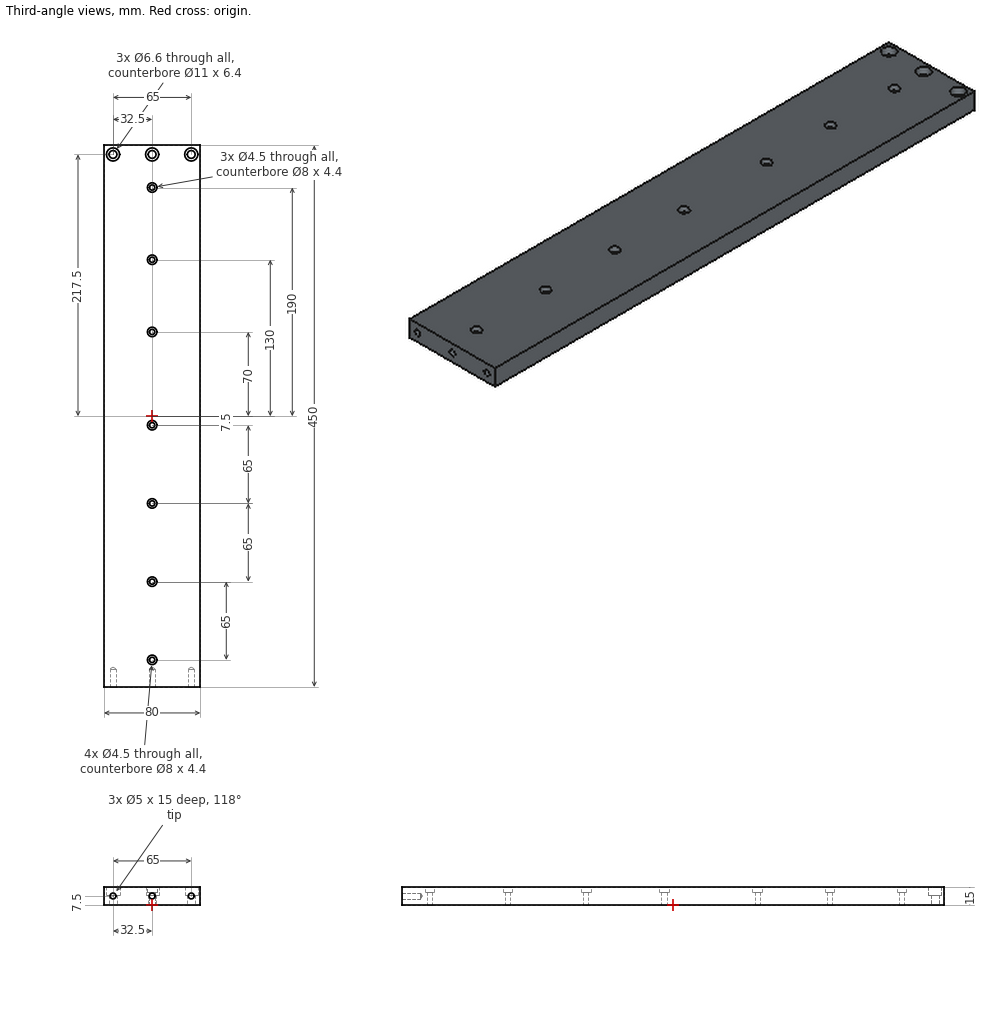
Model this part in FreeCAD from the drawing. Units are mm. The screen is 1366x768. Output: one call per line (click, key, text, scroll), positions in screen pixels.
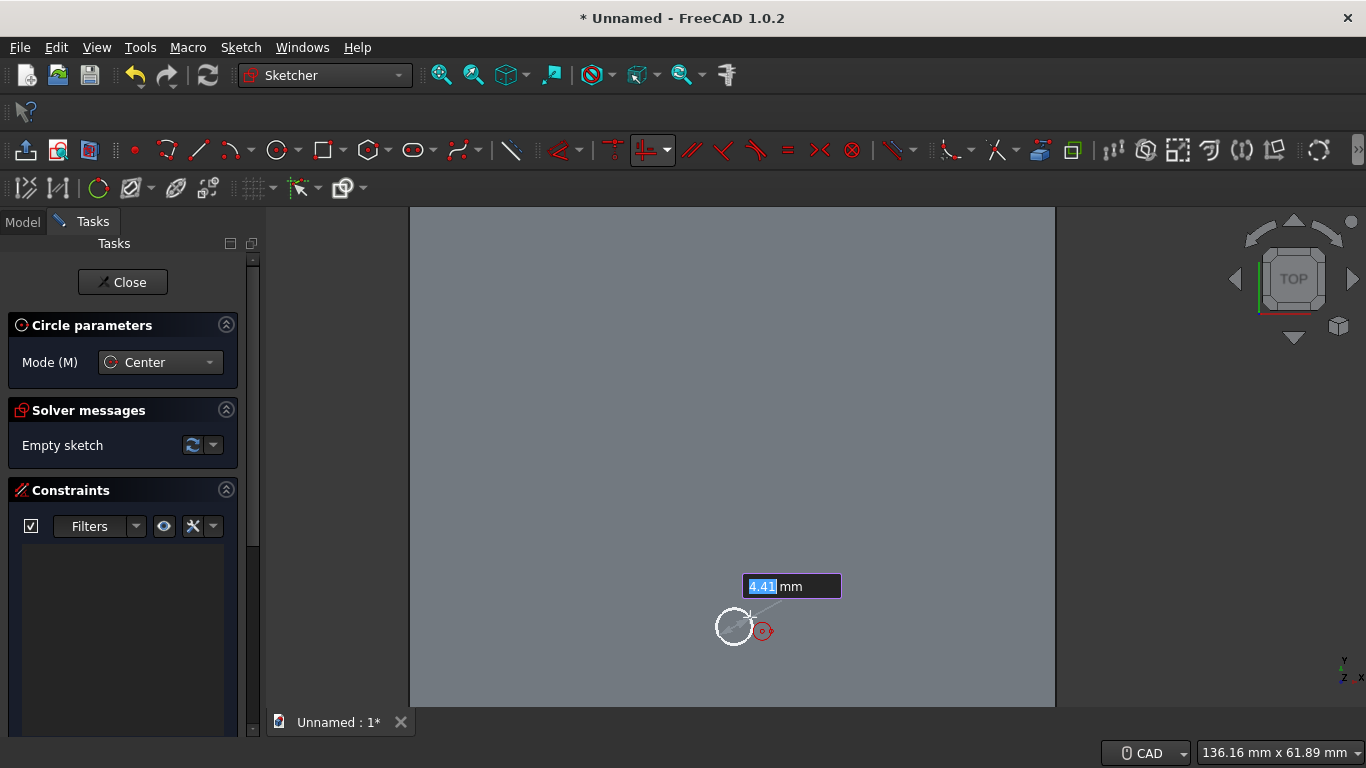
text(4.5)
key(Return)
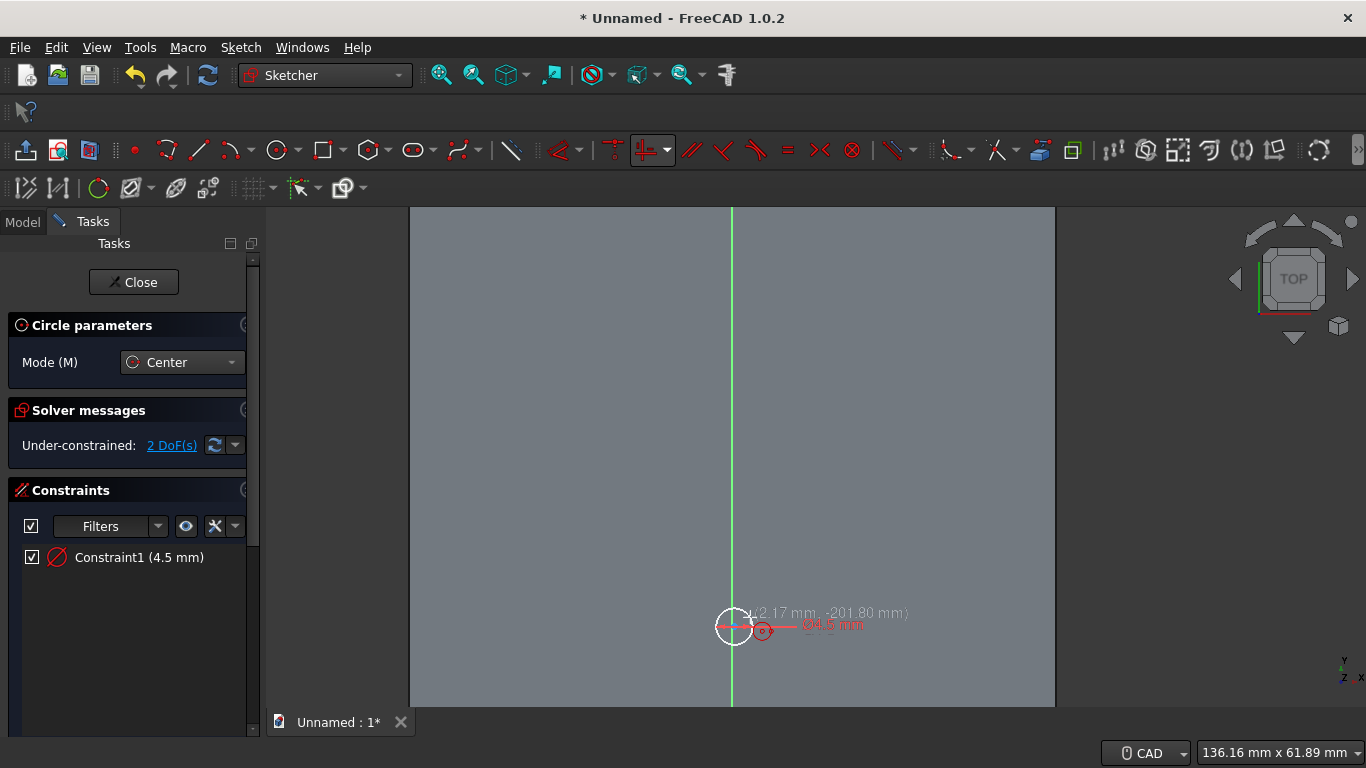
scroll(751, 619, down, 8)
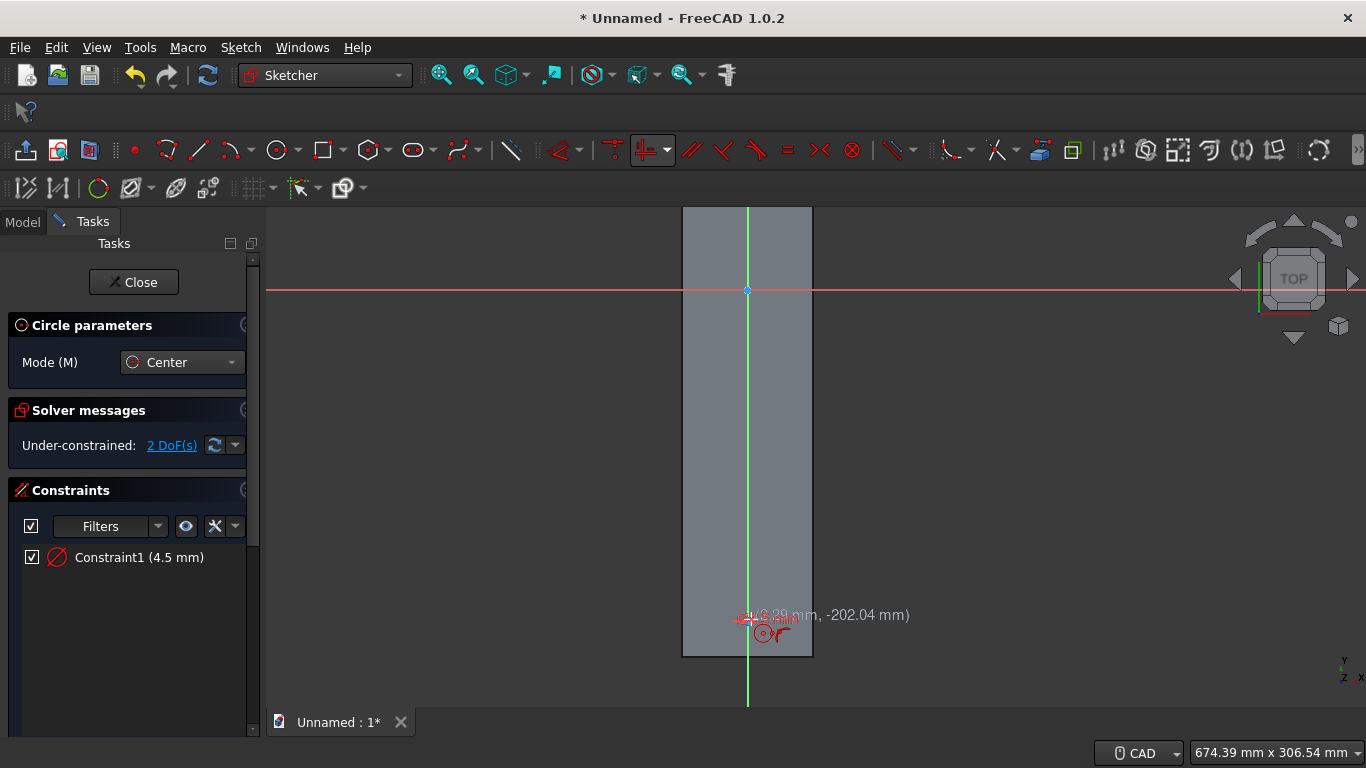
scroll(748, 515, up, 10)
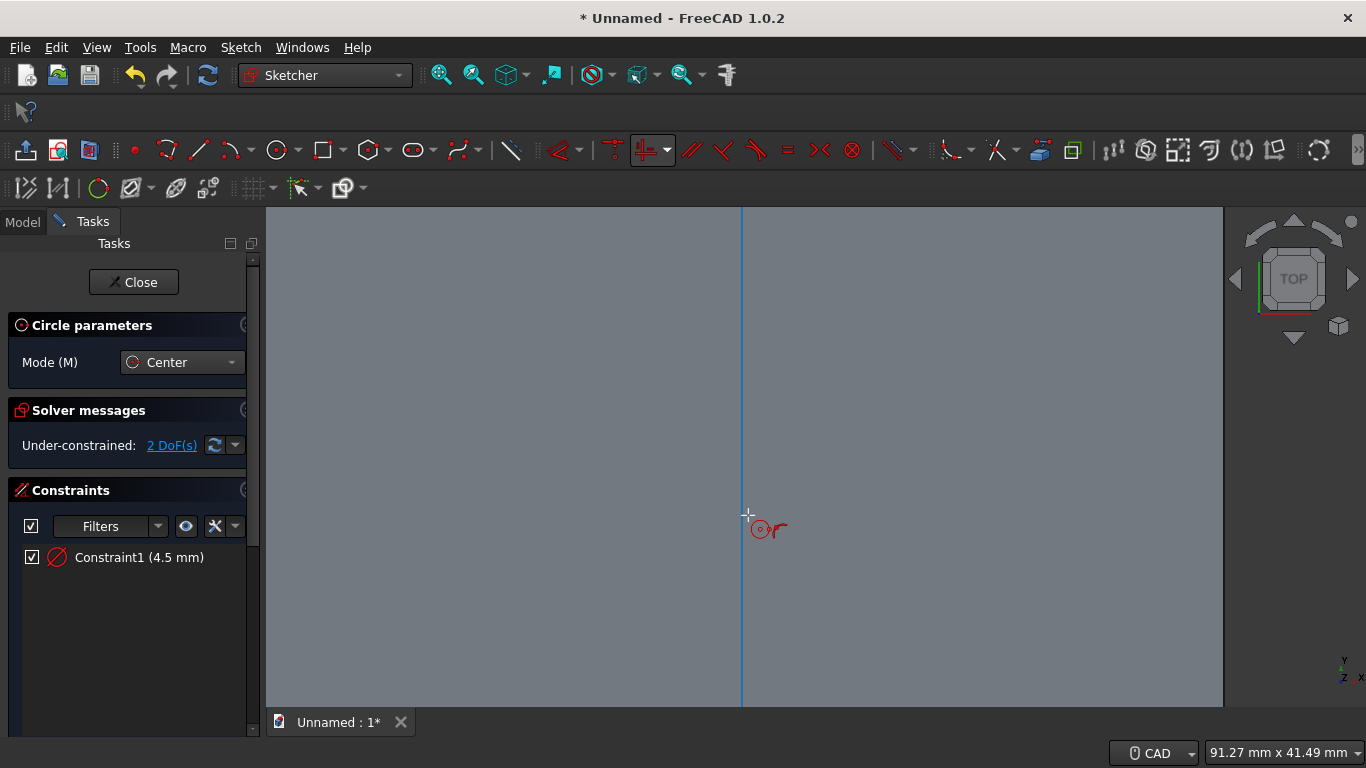
scroll(748, 515, down, 10)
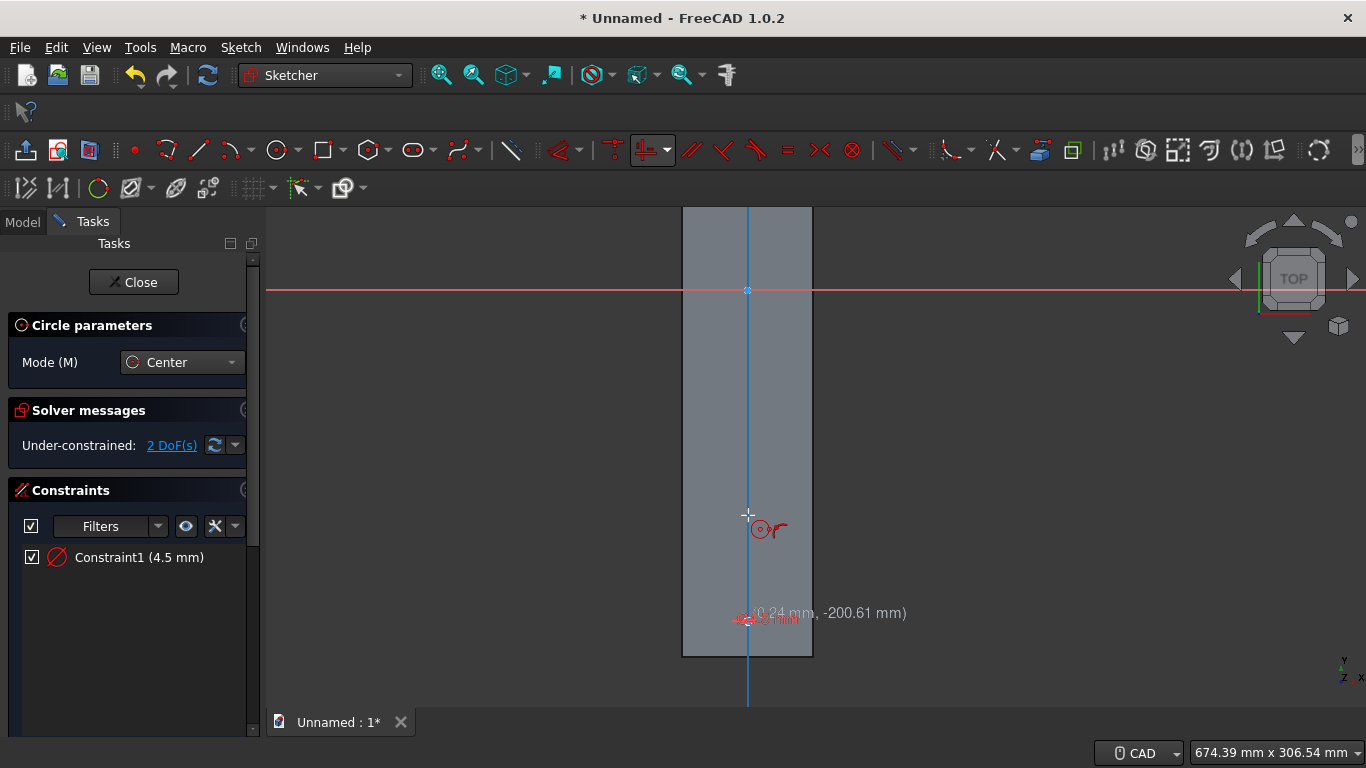
click(748, 515)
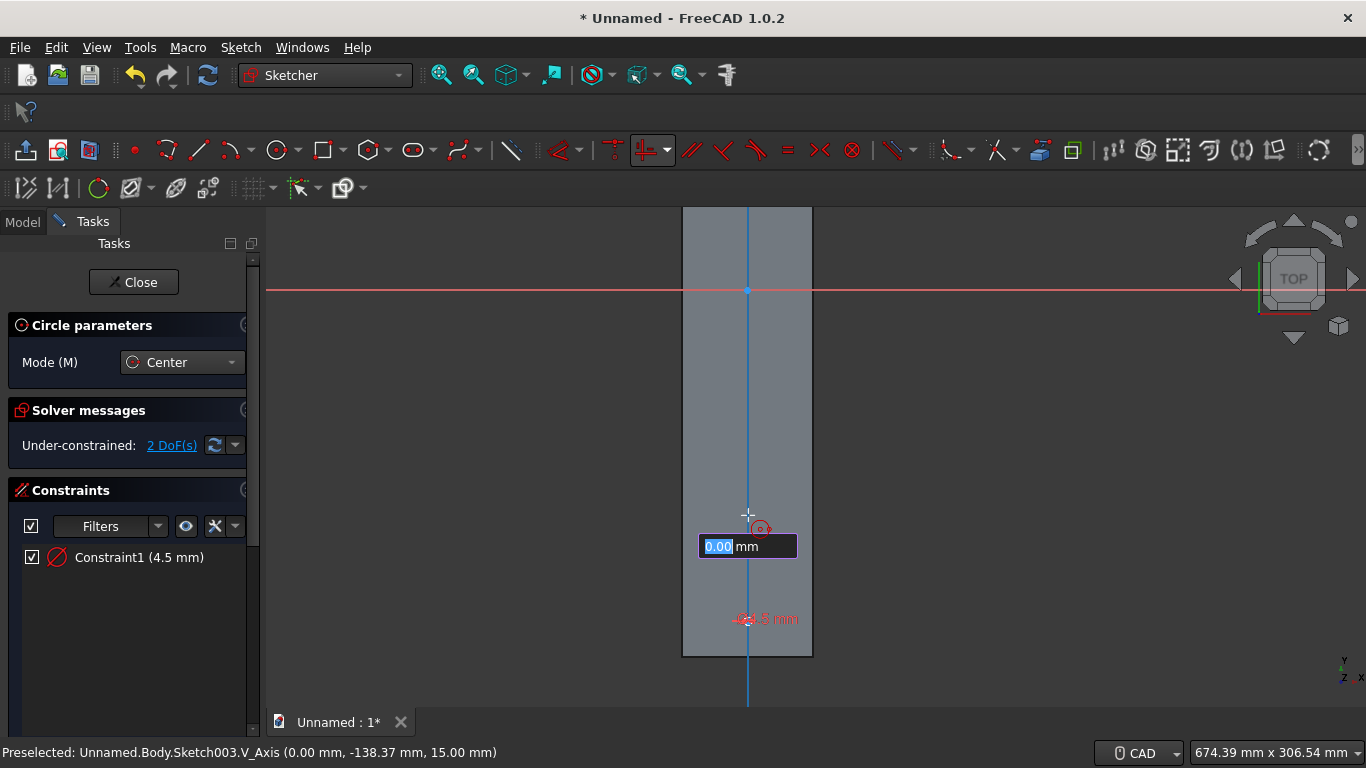
scroll(751, 513, up, 8)
move(750, 512)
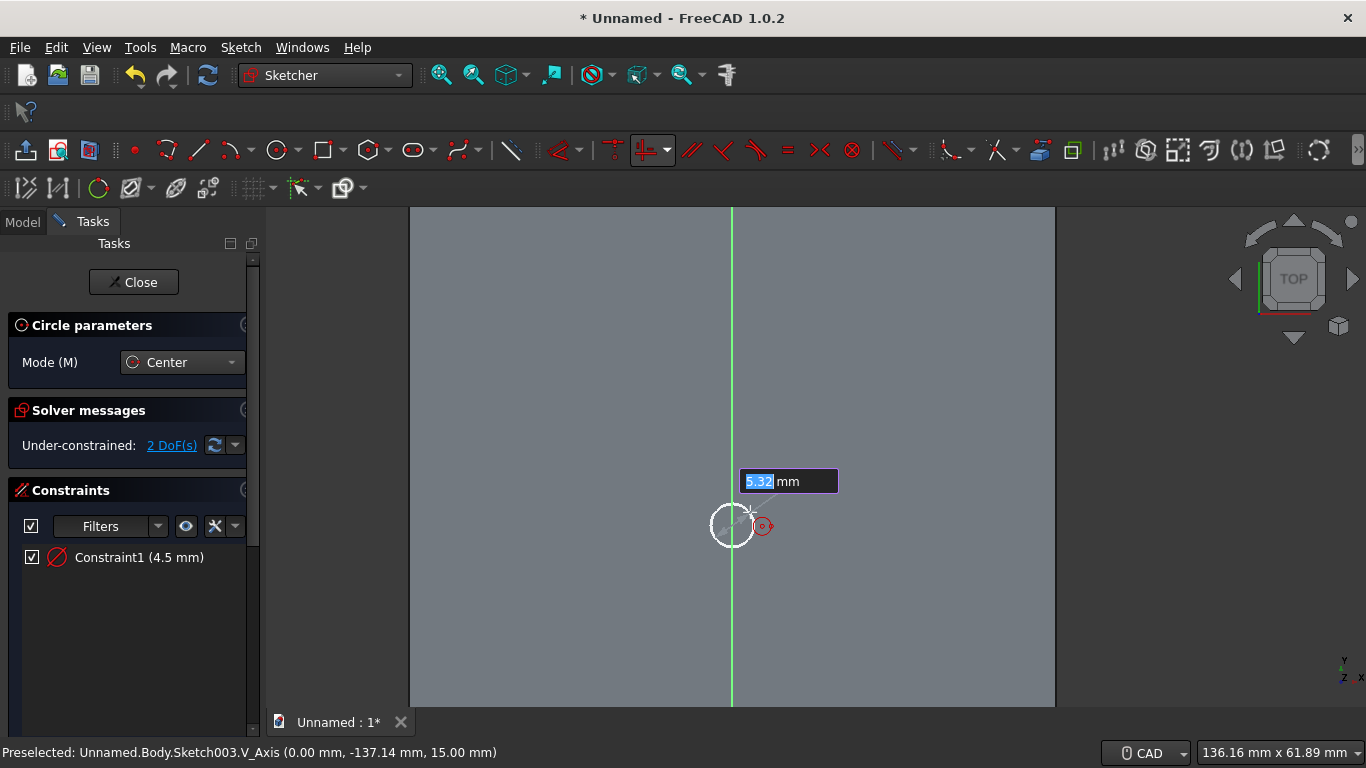
text(4.5)
key(Return)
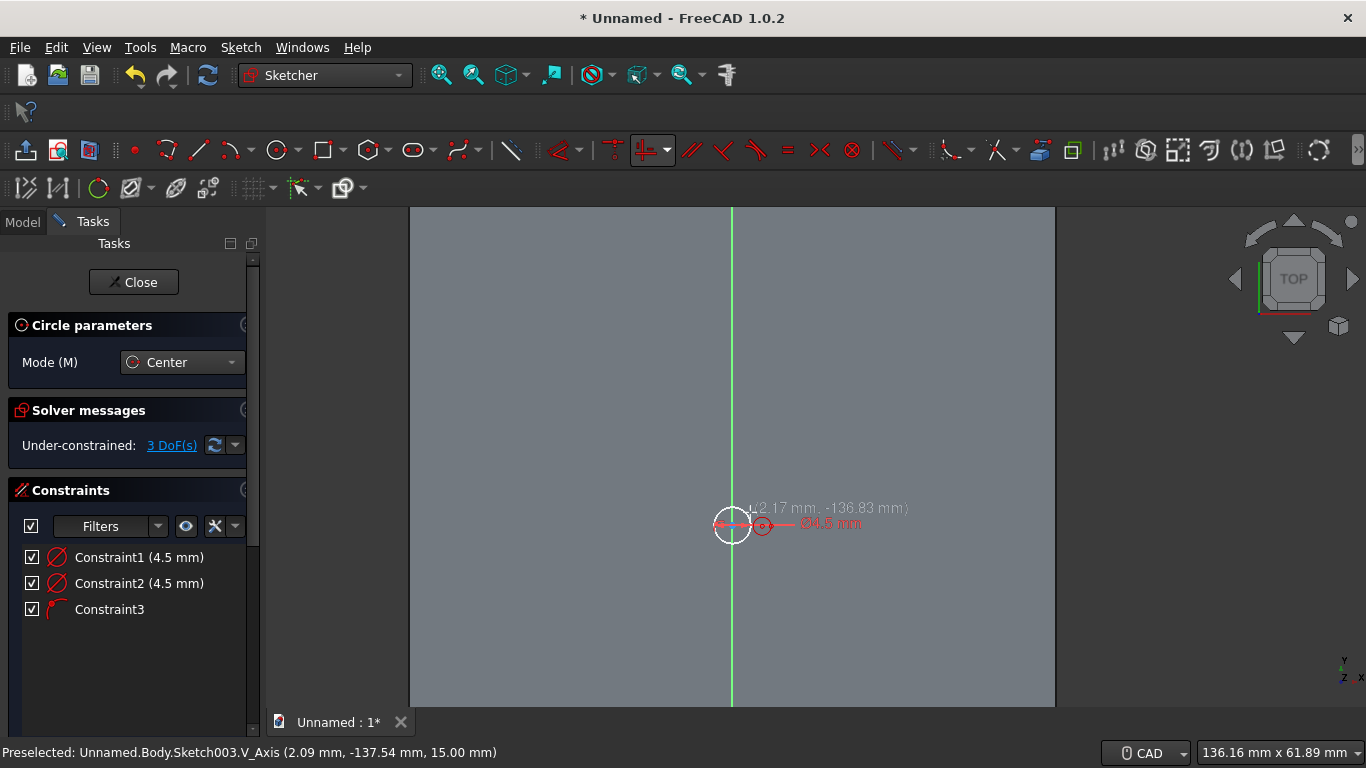
scroll(751, 513, down, 8)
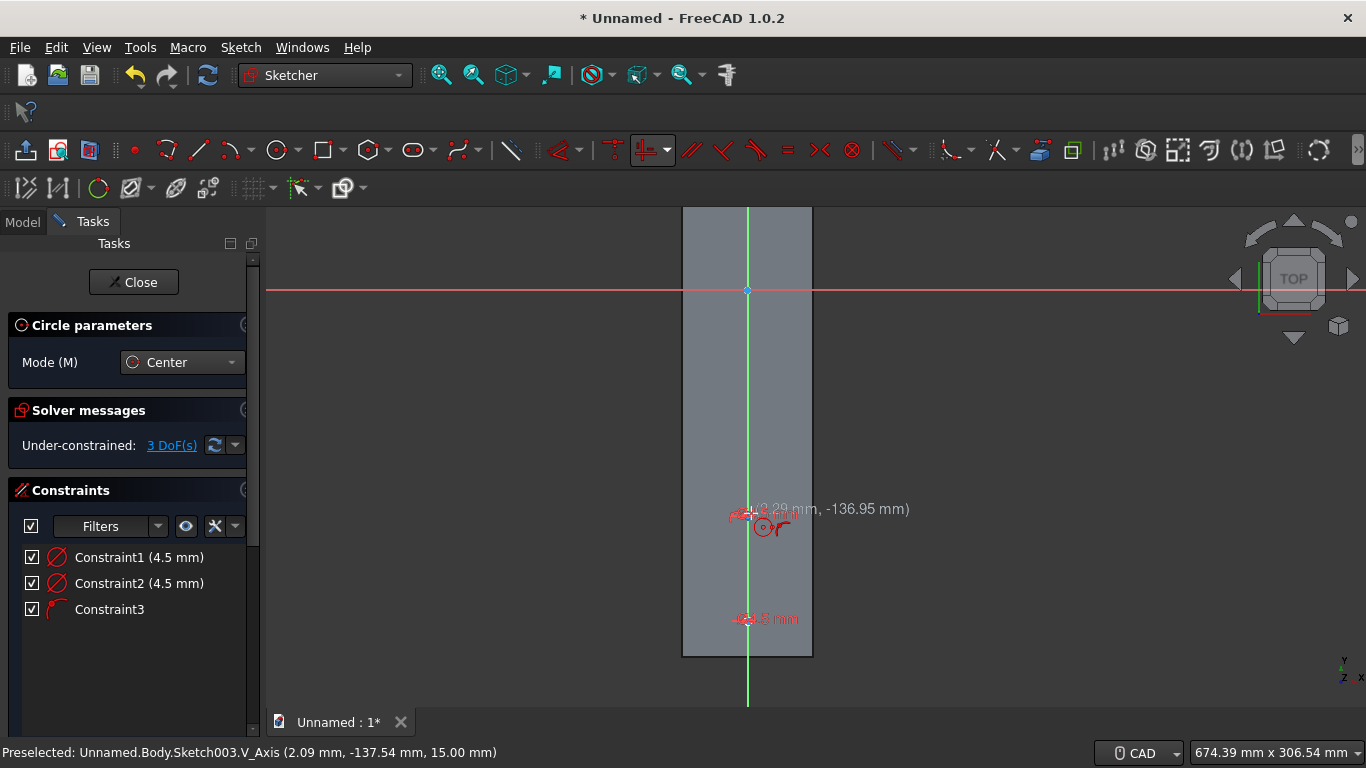
scroll(748, 409, up, 10)